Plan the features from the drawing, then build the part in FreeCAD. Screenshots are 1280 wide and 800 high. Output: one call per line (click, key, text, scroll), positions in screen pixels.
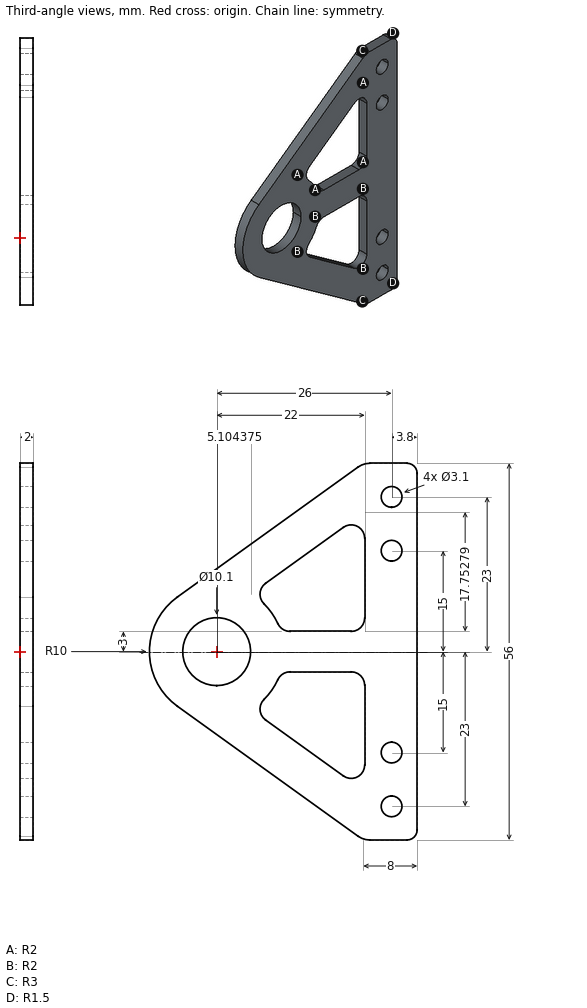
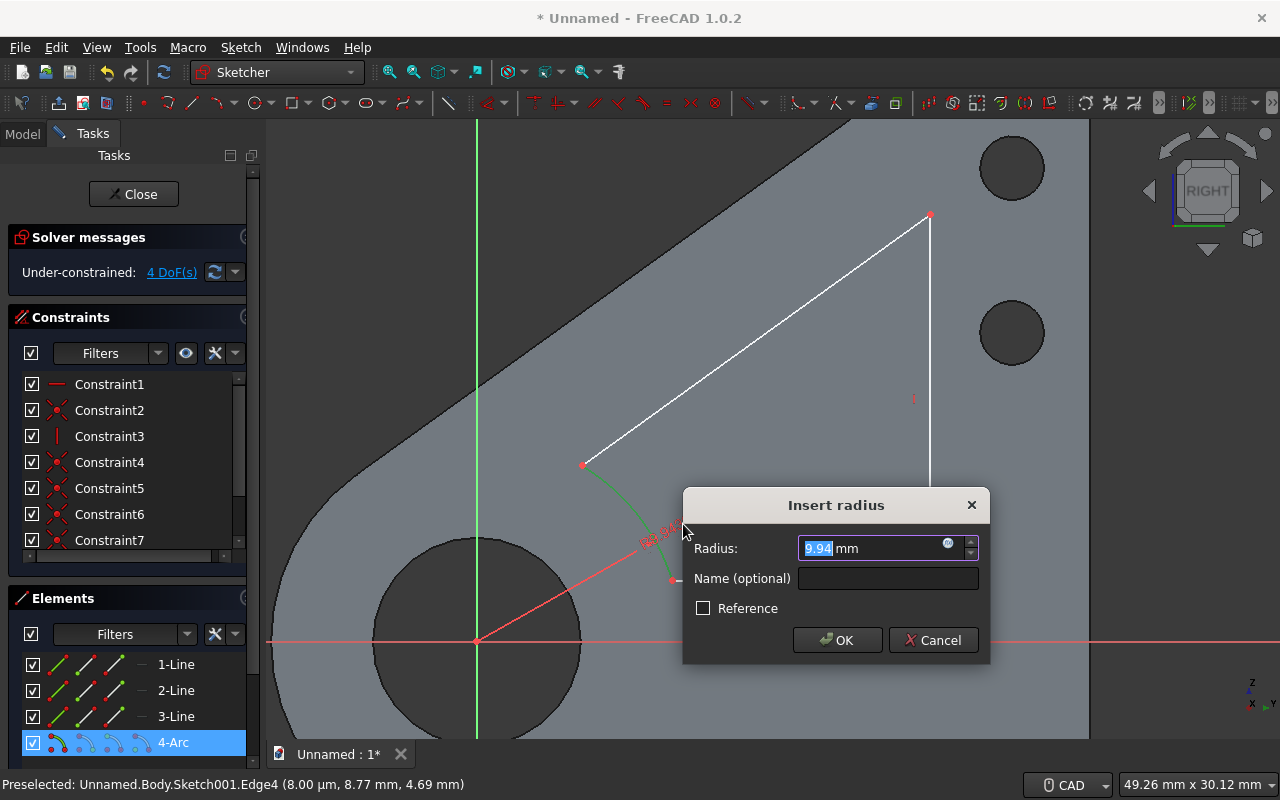
text(10)
key(Return)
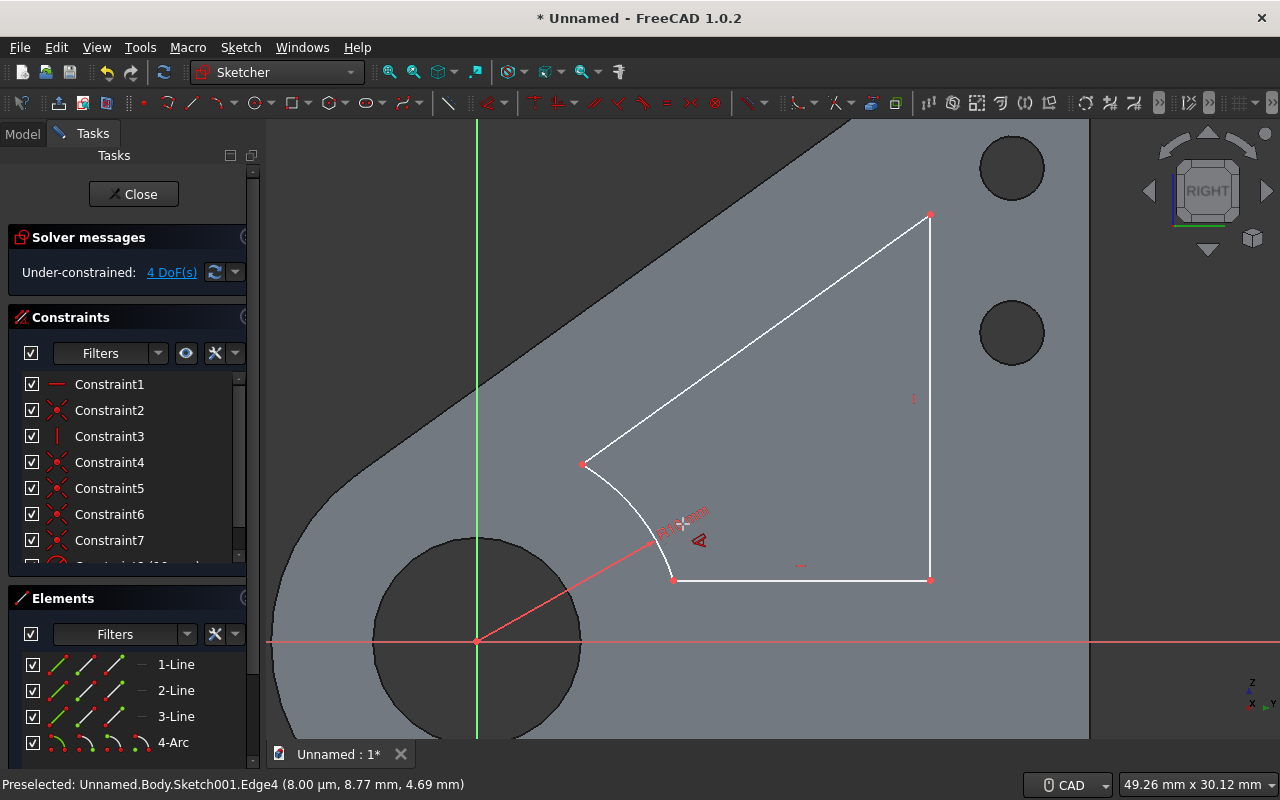
click(674, 581)
click(443, 611)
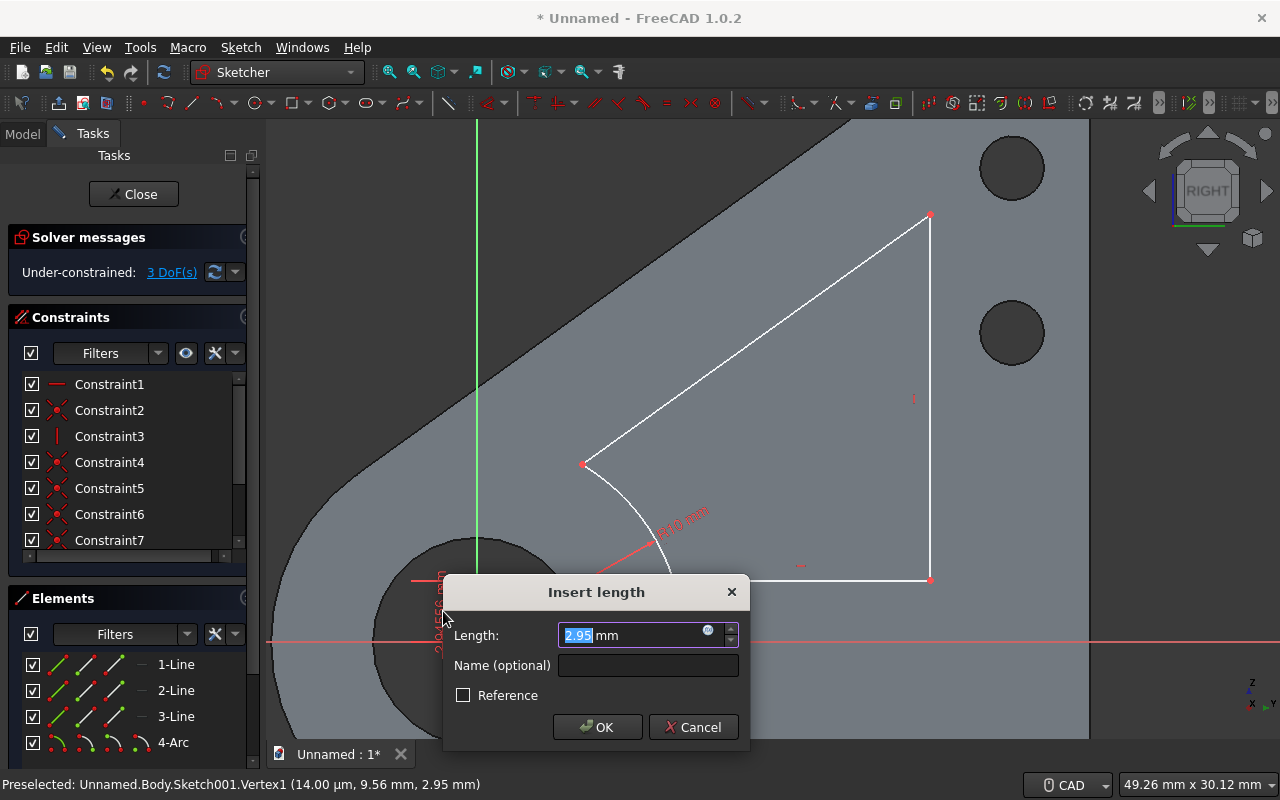
text(3)
key(Return)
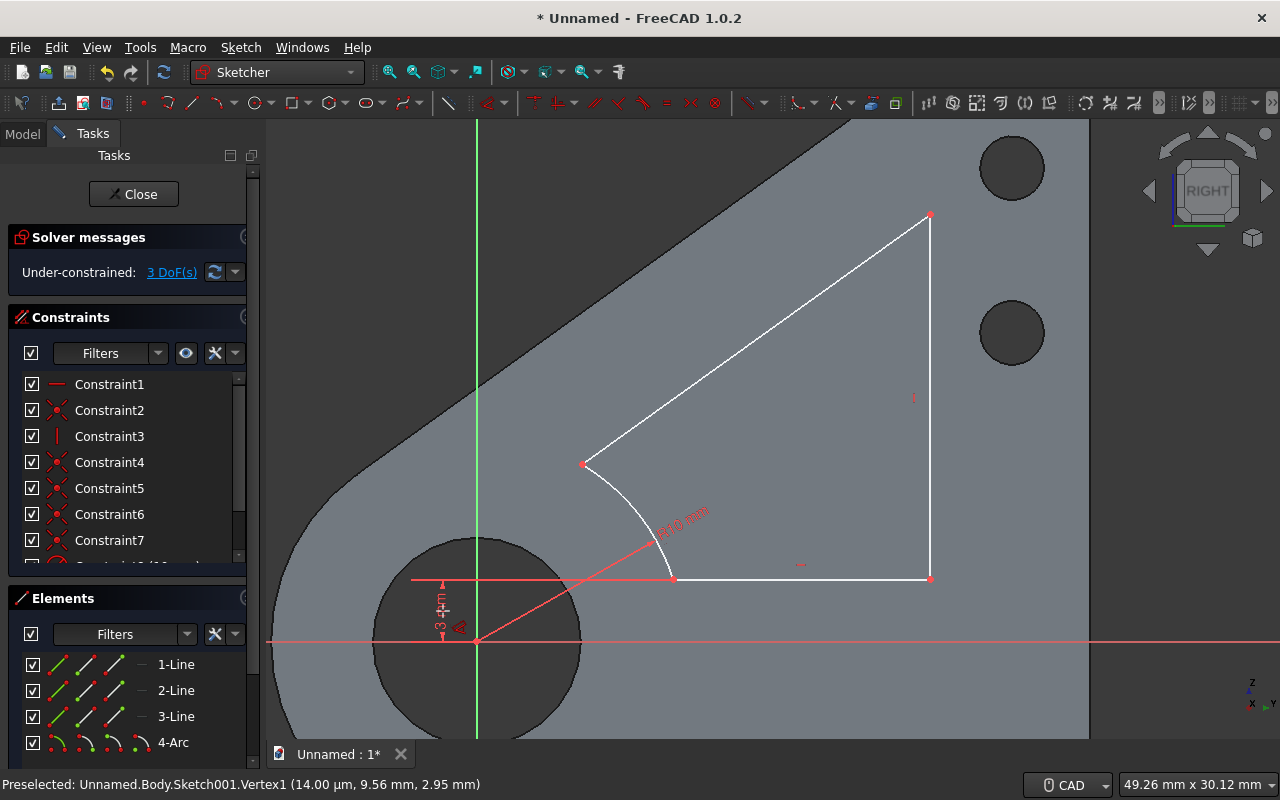
click(930, 580)
click(703, 676)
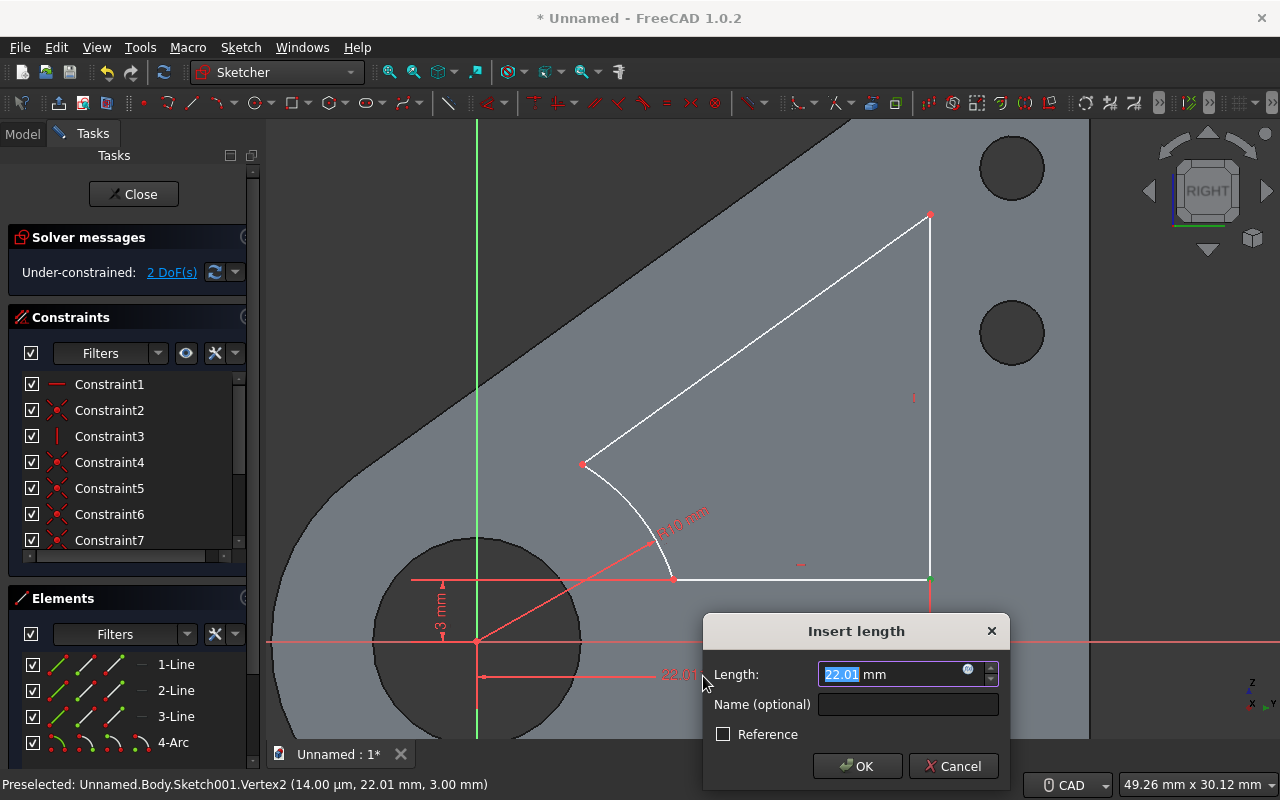
text(22)
key(Return)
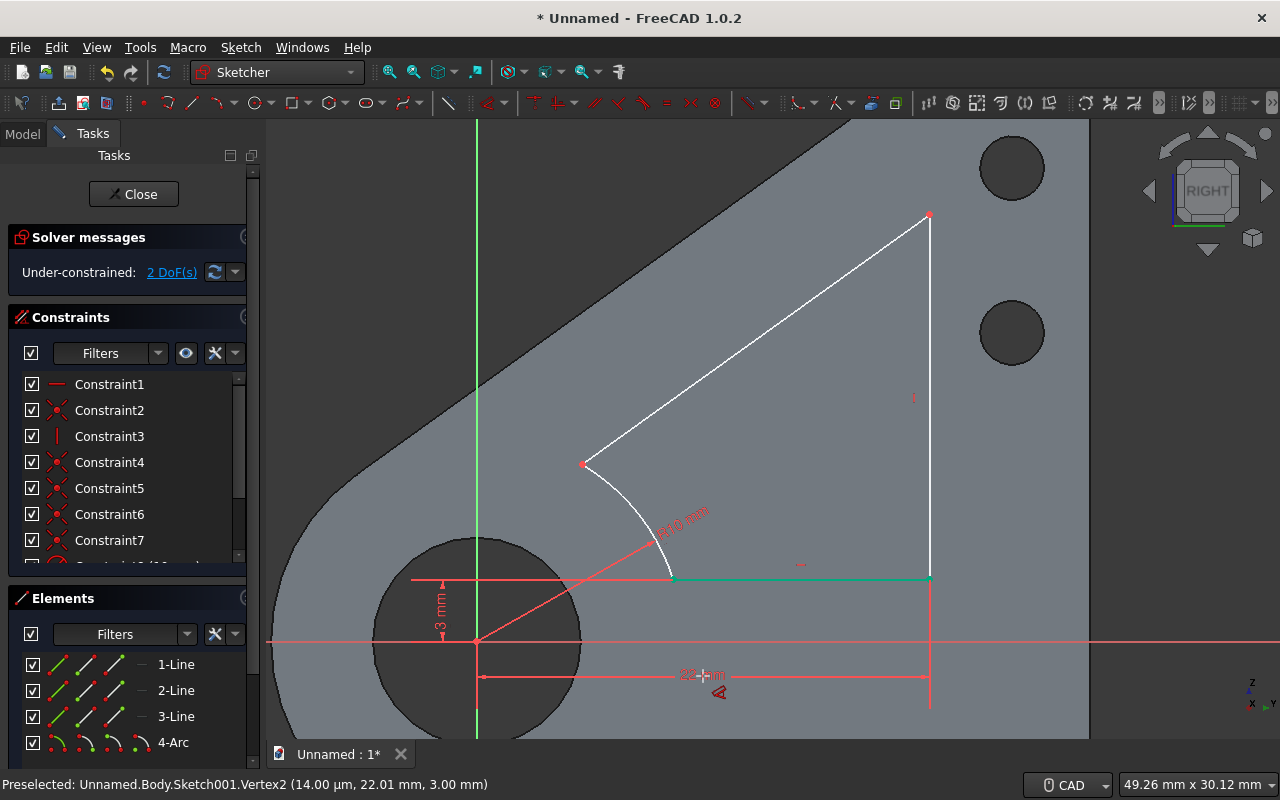
click(930, 470)
click(964, 397)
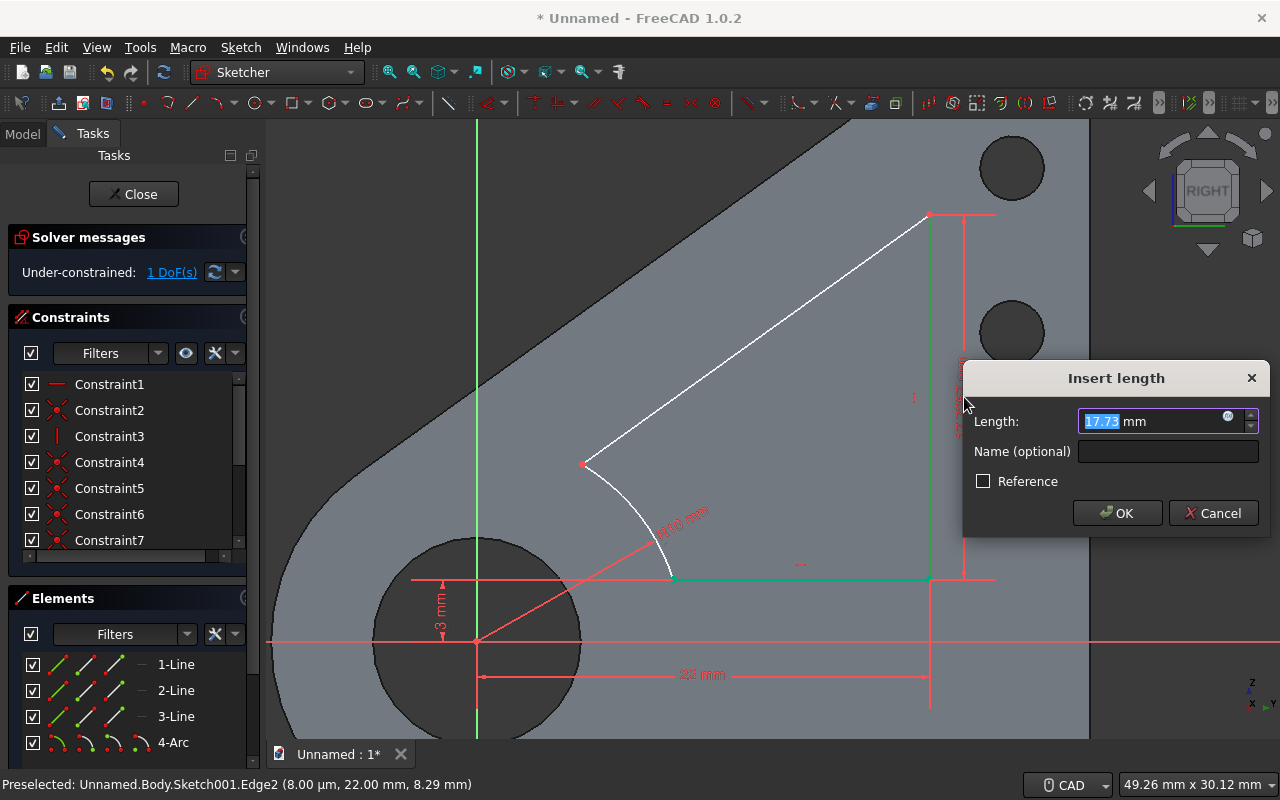
text(17.75279)
key(Return)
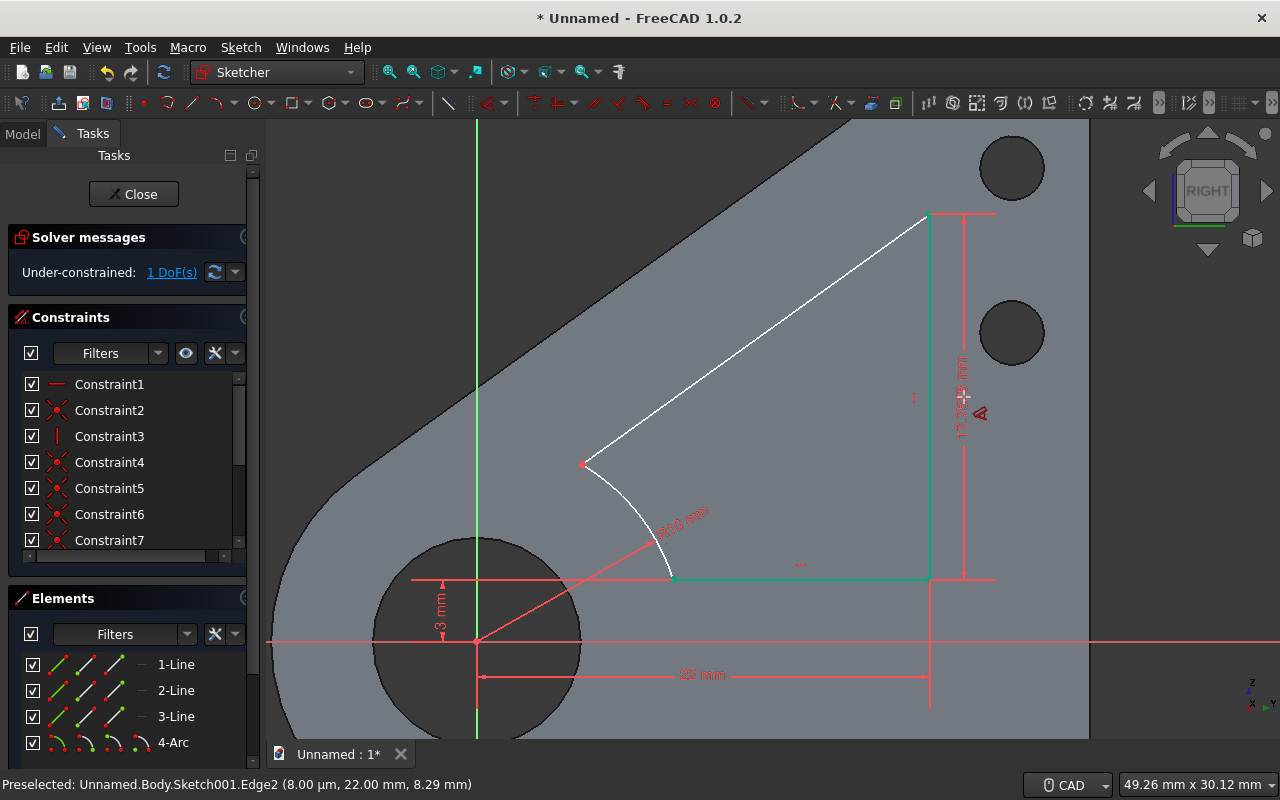
click(582, 465)
click(529, 676)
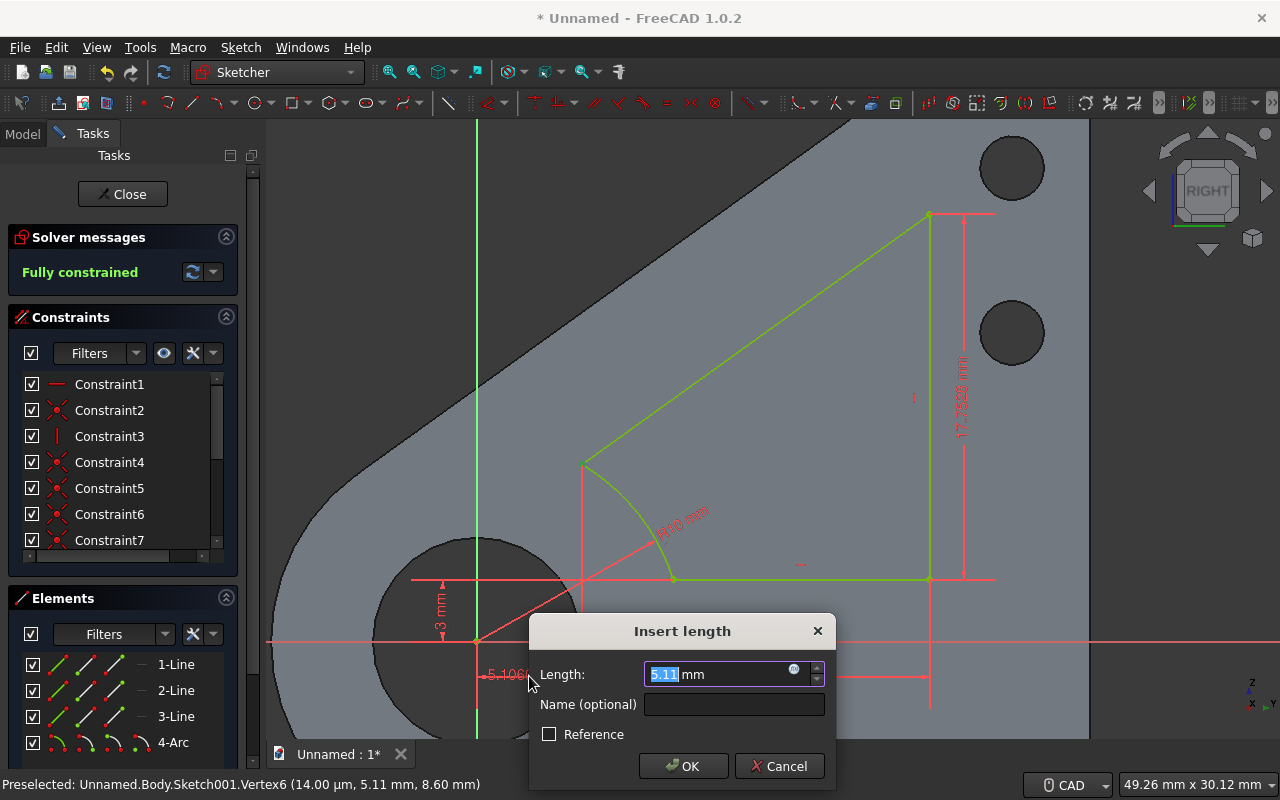
text(5.104375)
key(Return)
key(Escape)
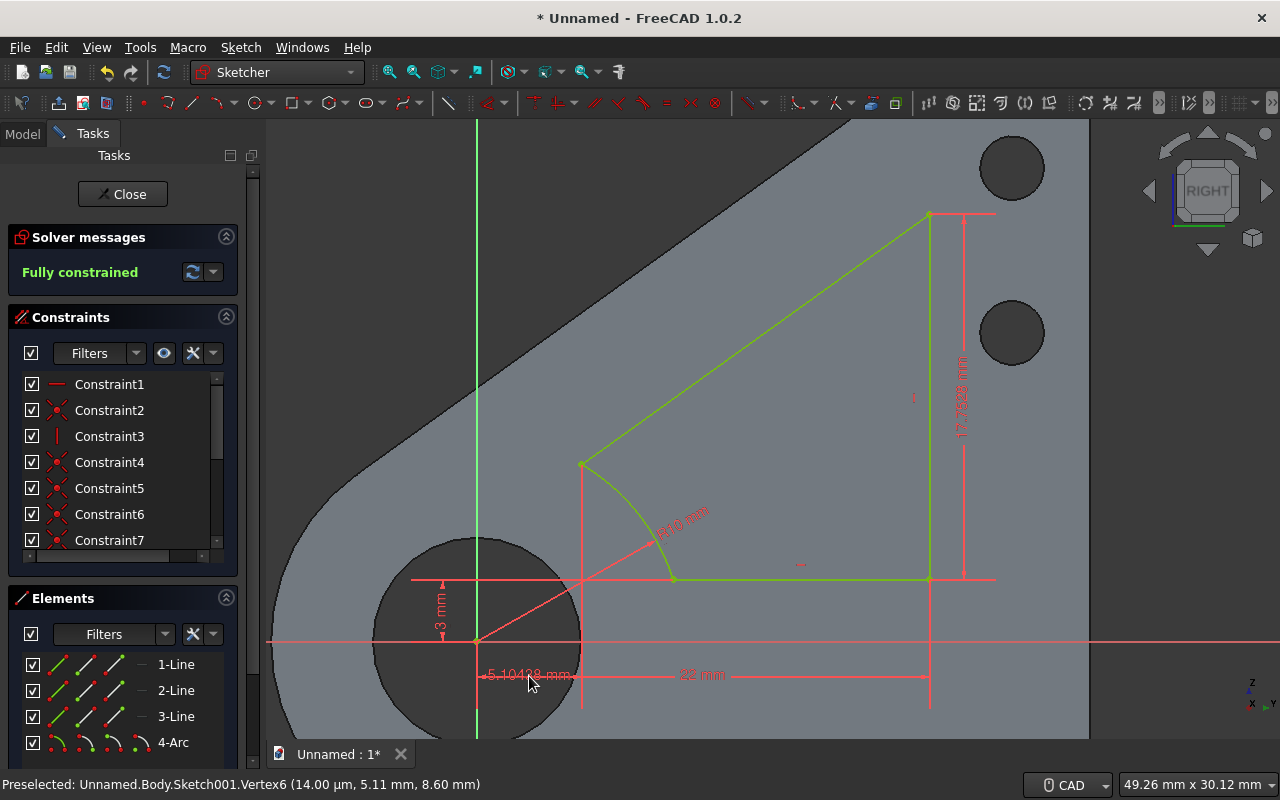
click(123, 194)